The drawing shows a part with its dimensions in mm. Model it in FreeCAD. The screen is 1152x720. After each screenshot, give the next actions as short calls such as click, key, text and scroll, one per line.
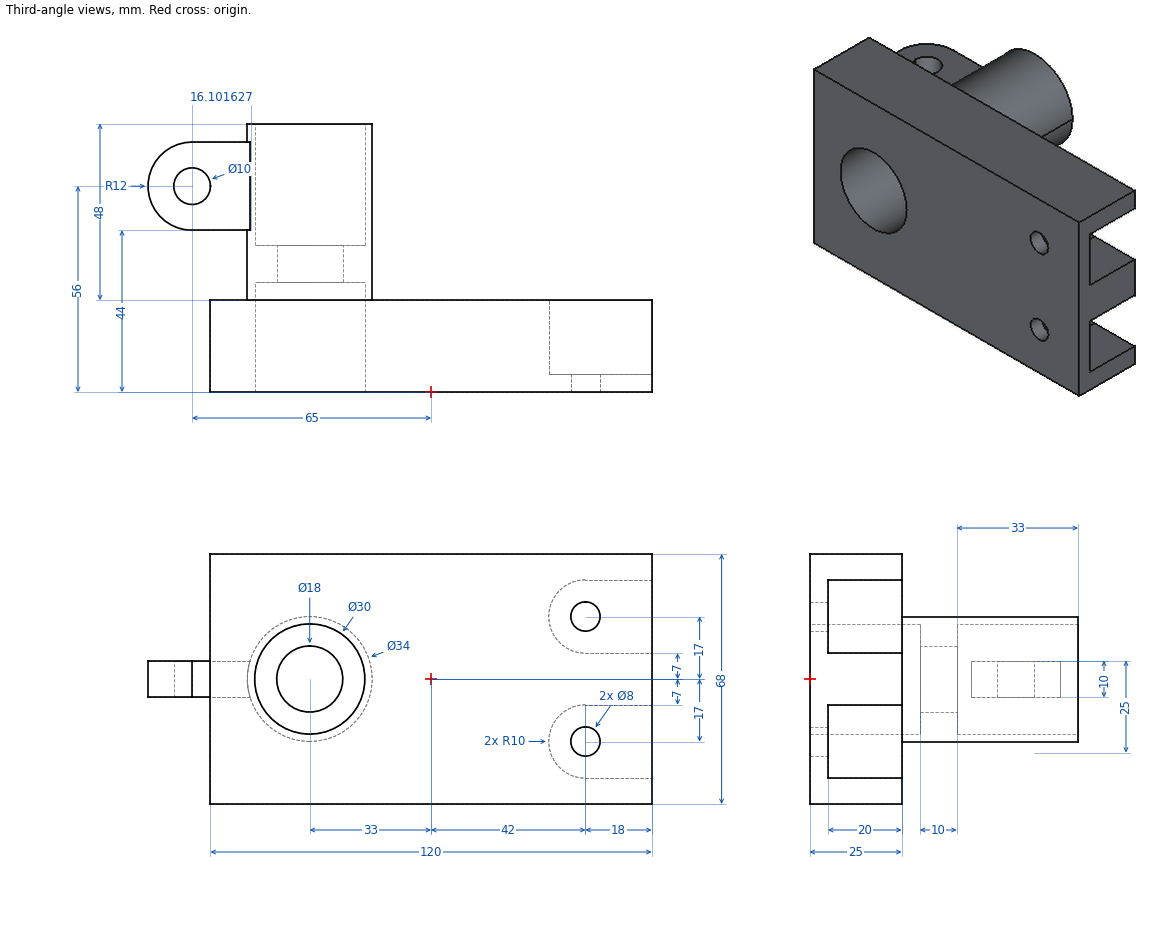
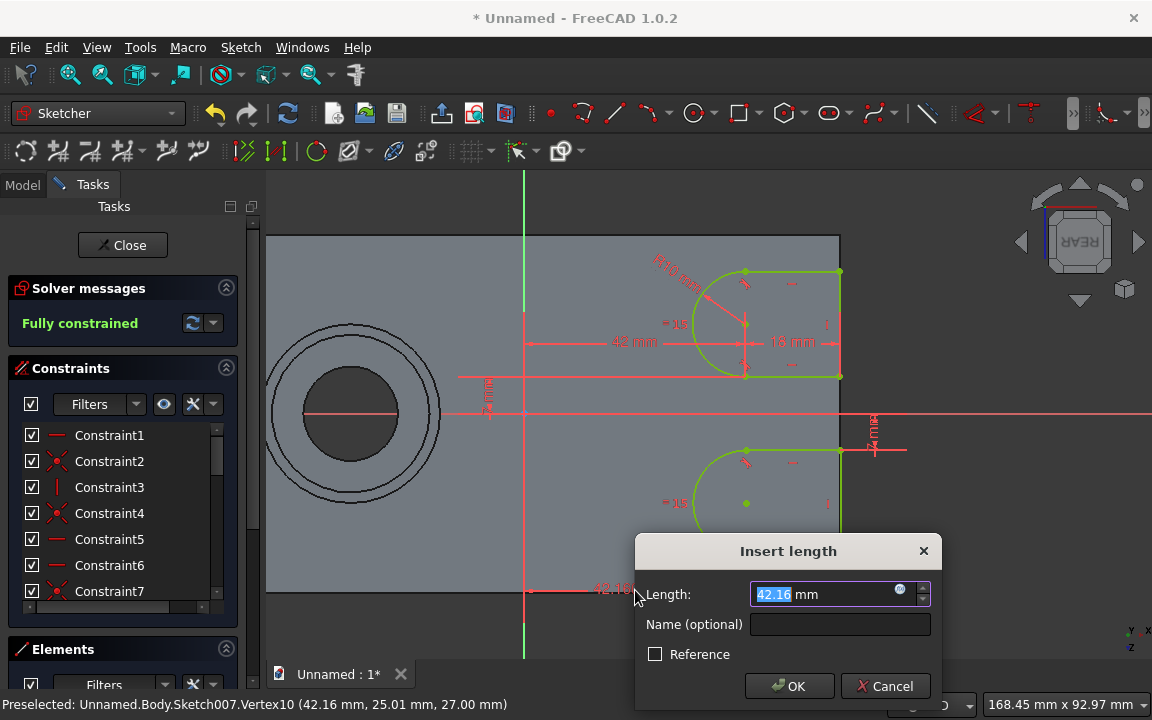
text(42)
key(Return)
key(Escape)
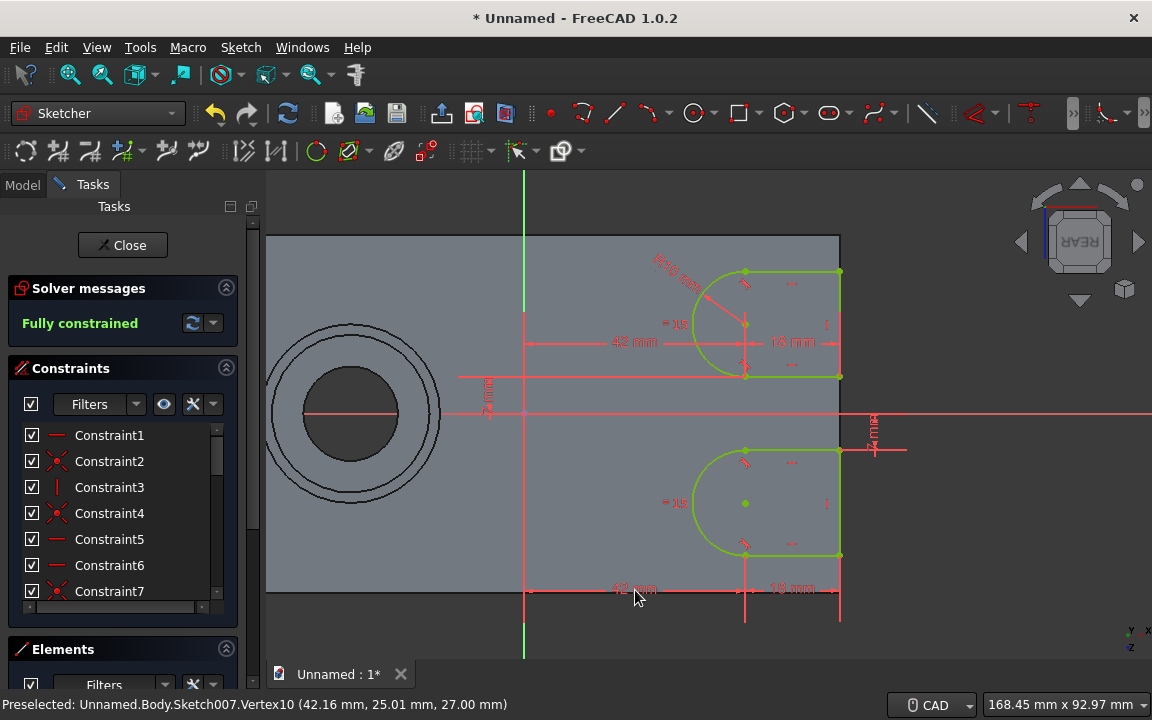
click(123, 245)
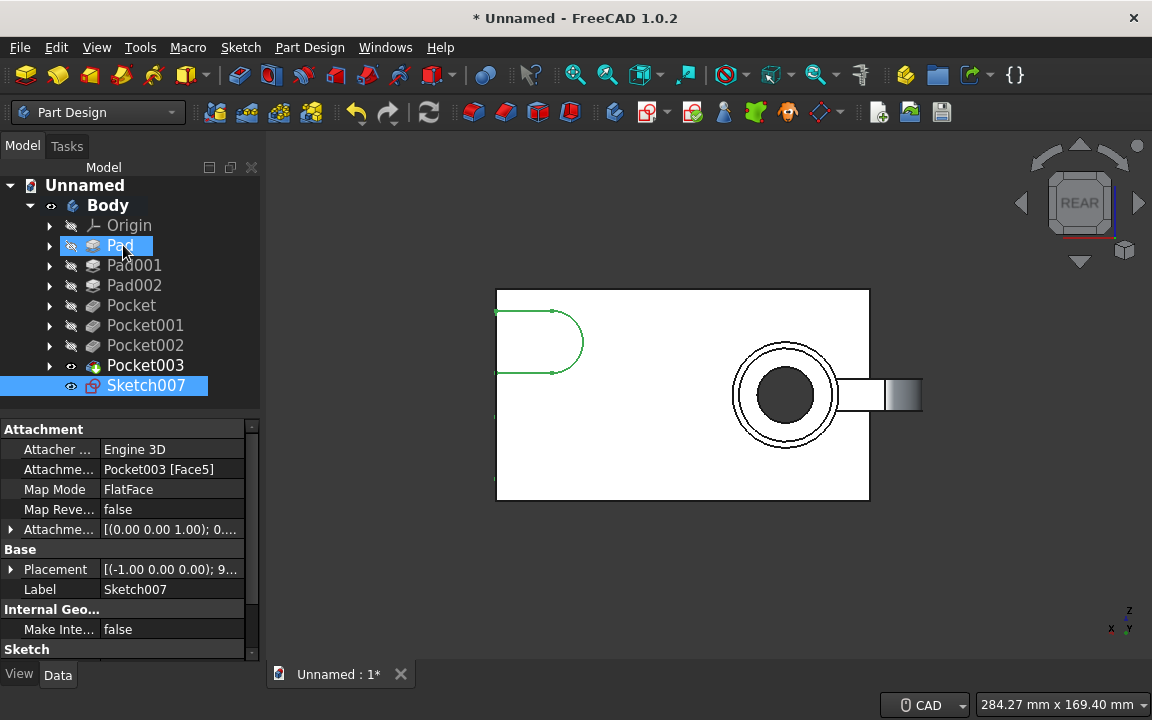
click(240, 76)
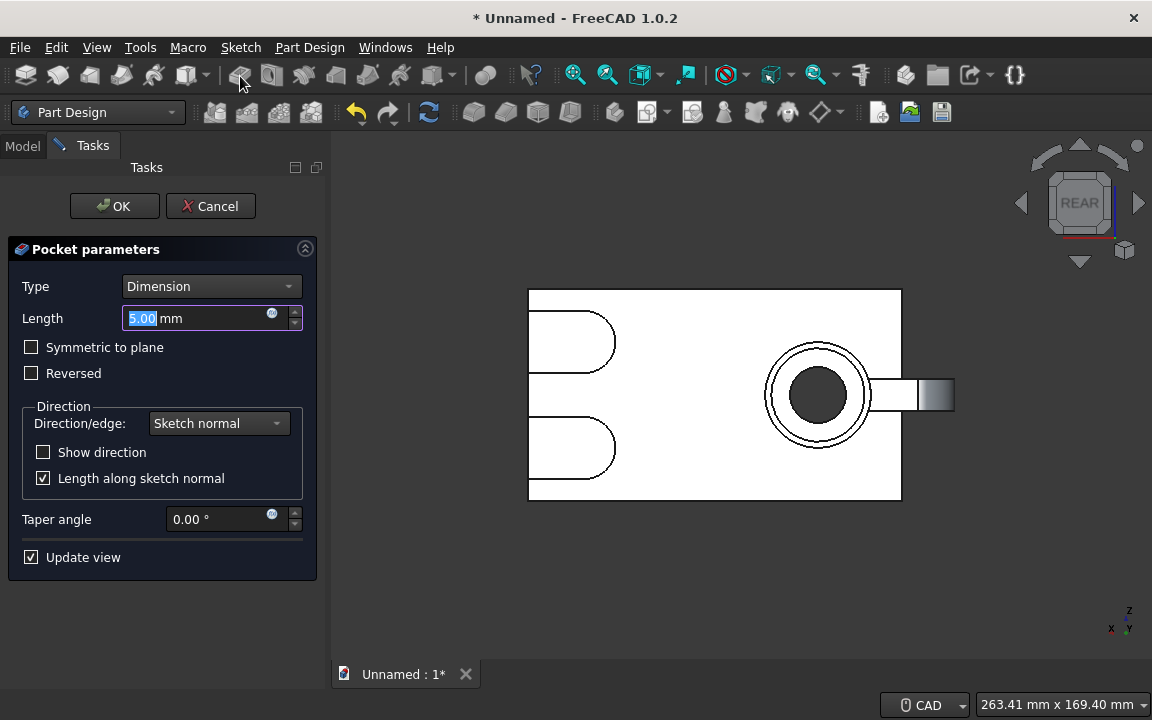
text(20)
key(Tab)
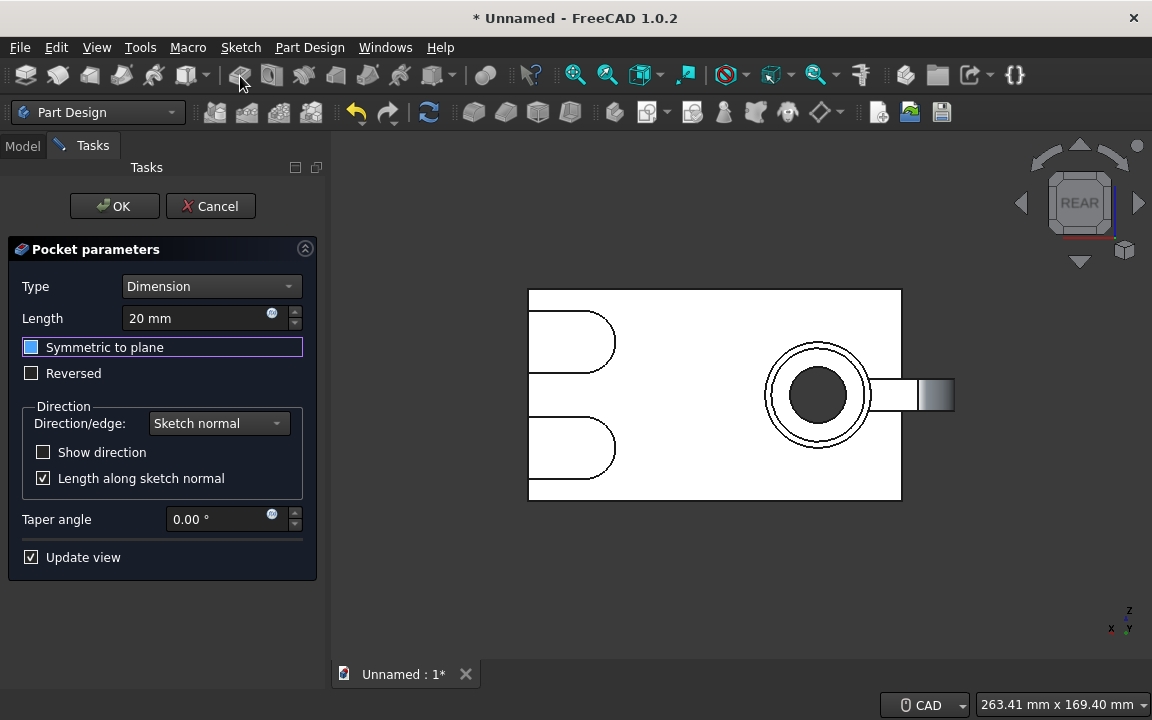
click(115, 206)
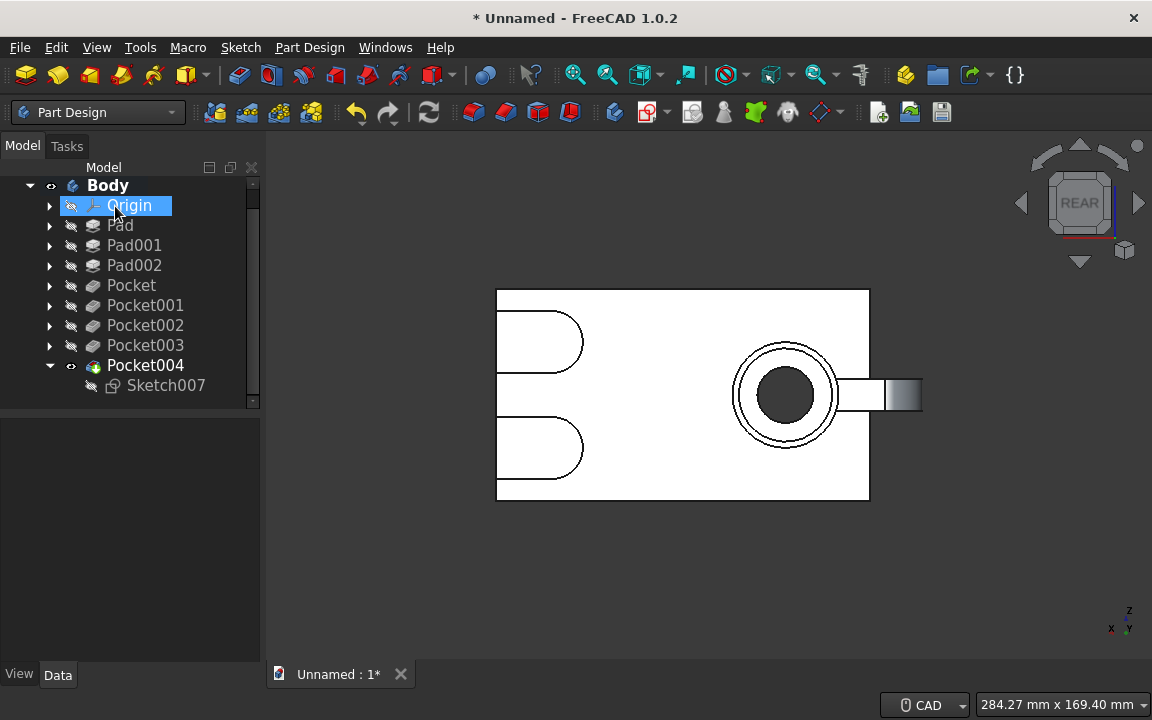
click(539, 341)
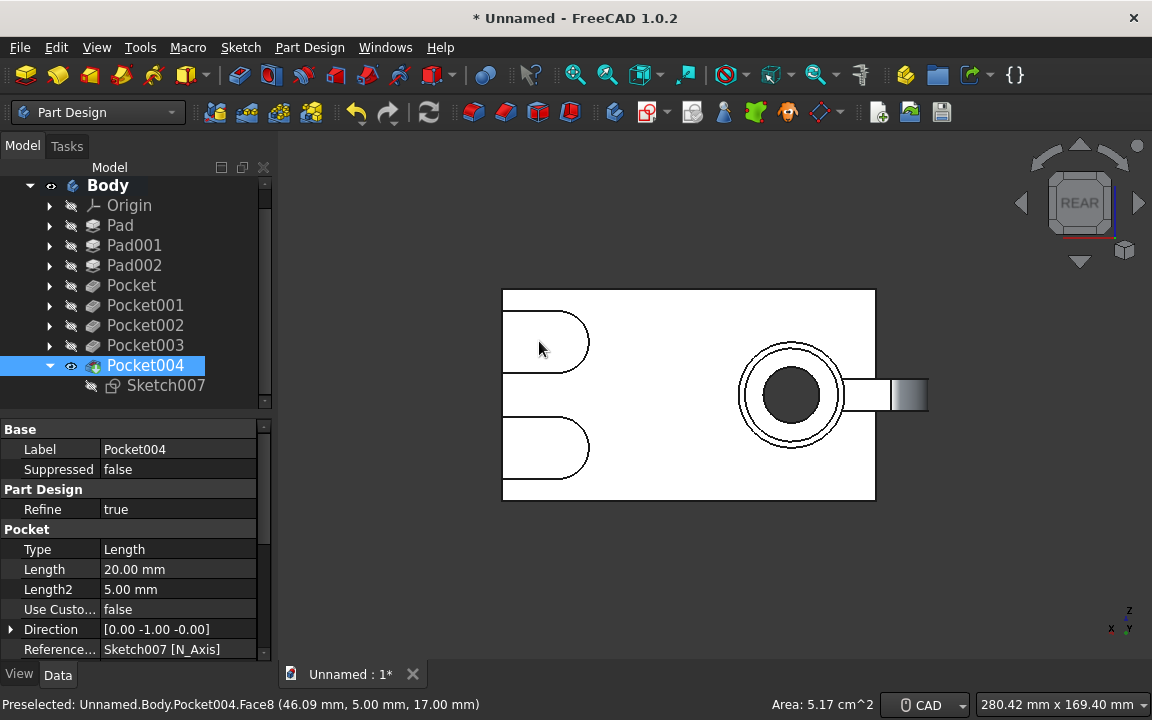
click(648, 112)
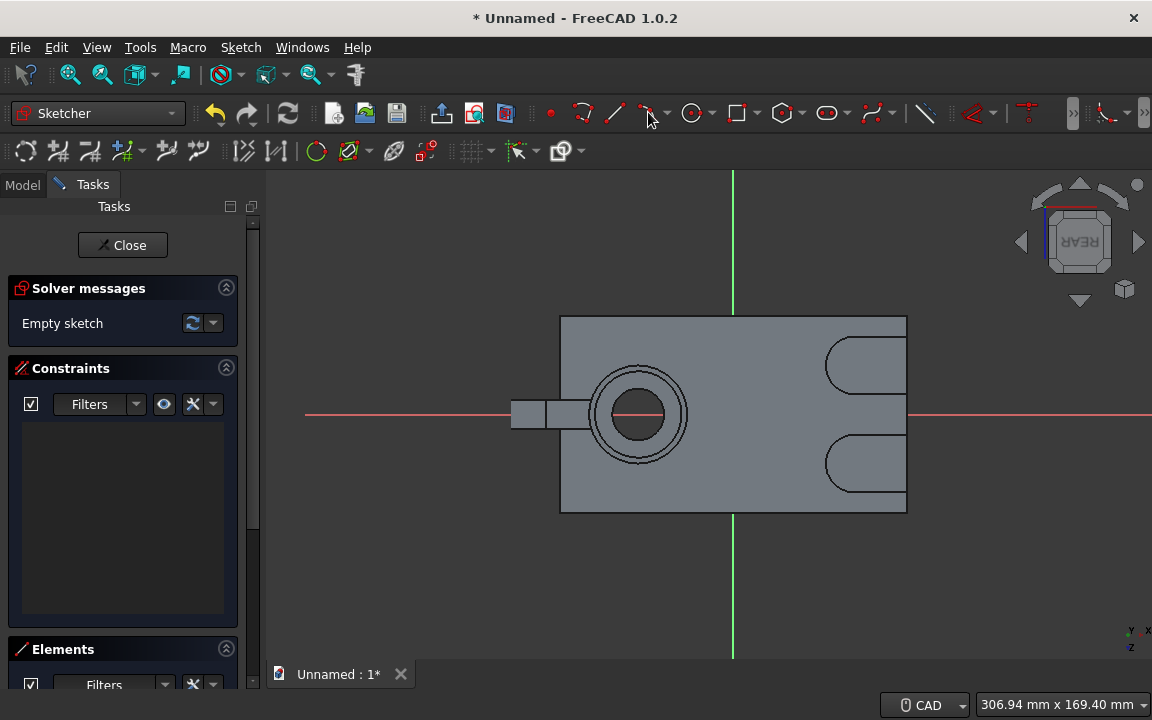
scroll(893, 414, up, 5)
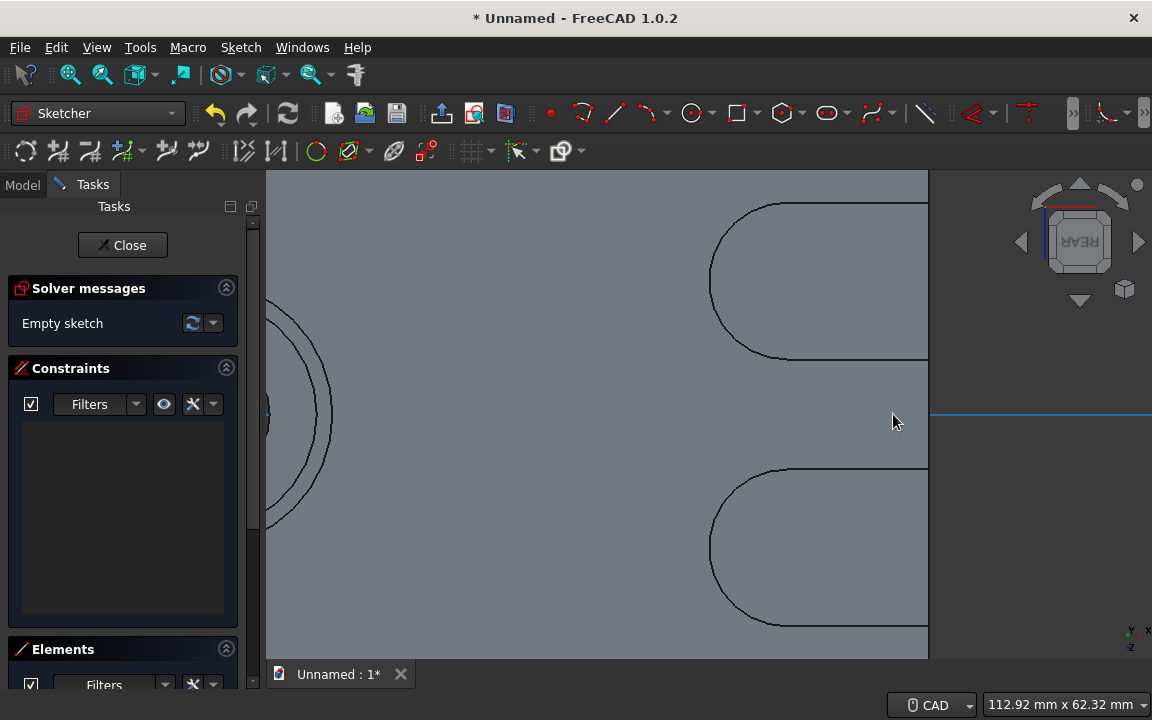
click(692, 114)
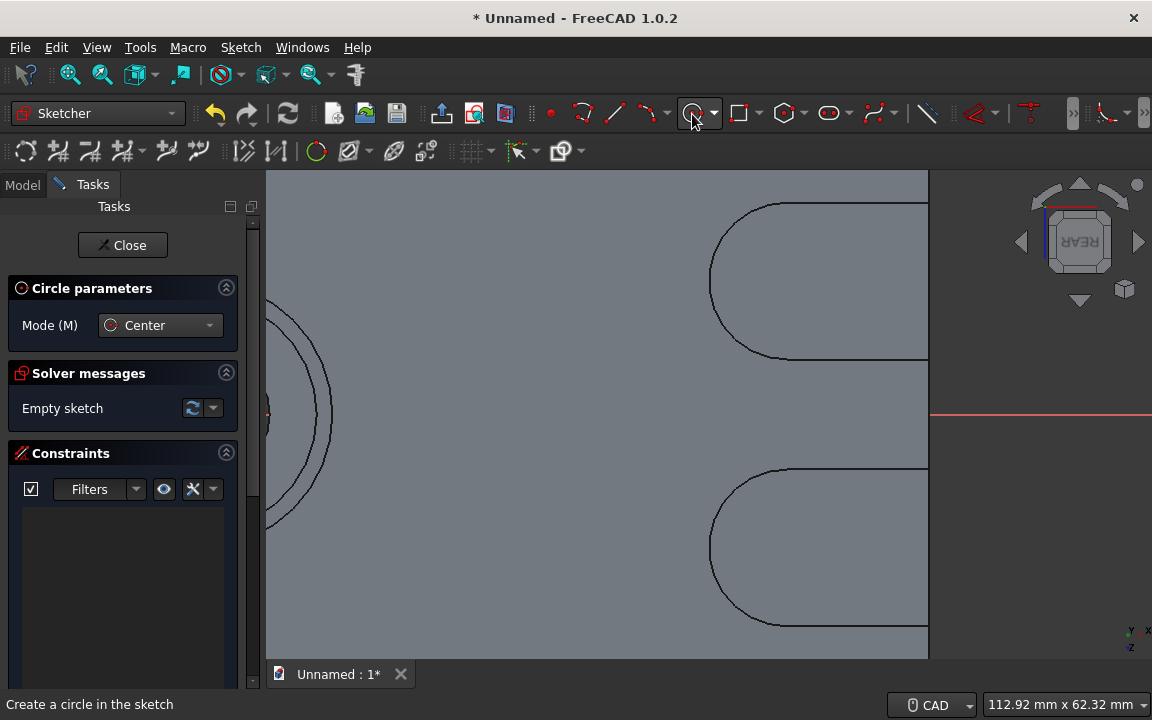
click(788, 281)
move(810, 259)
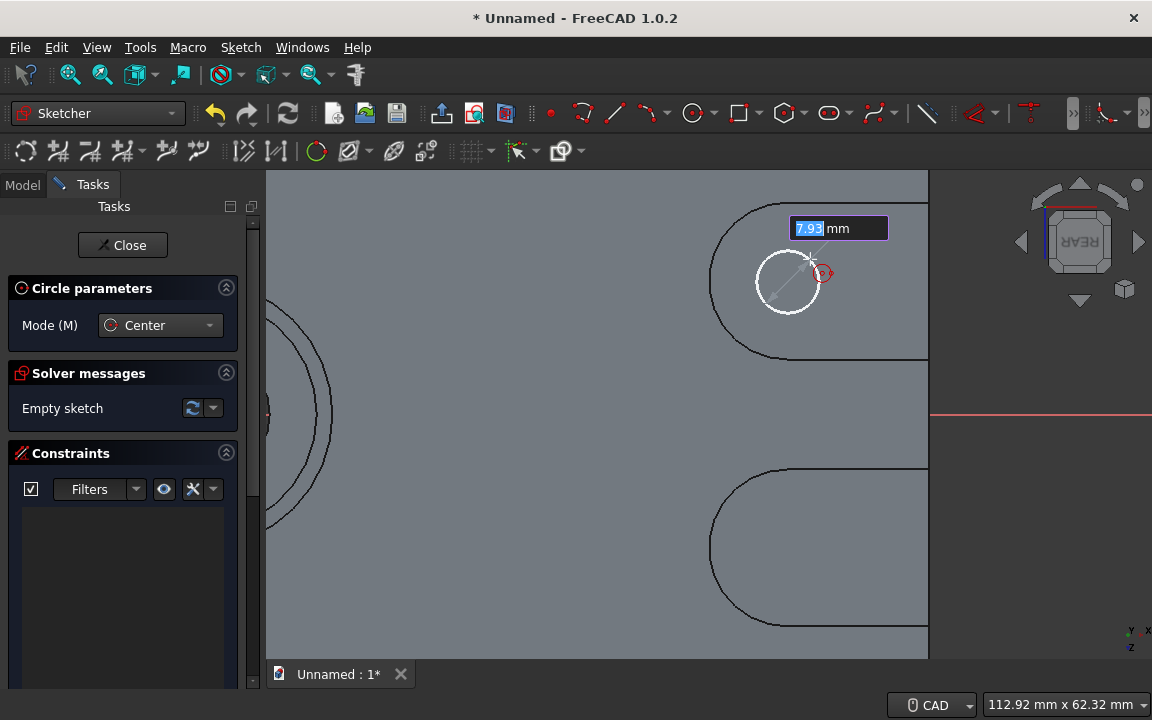
text(8)
key(Return)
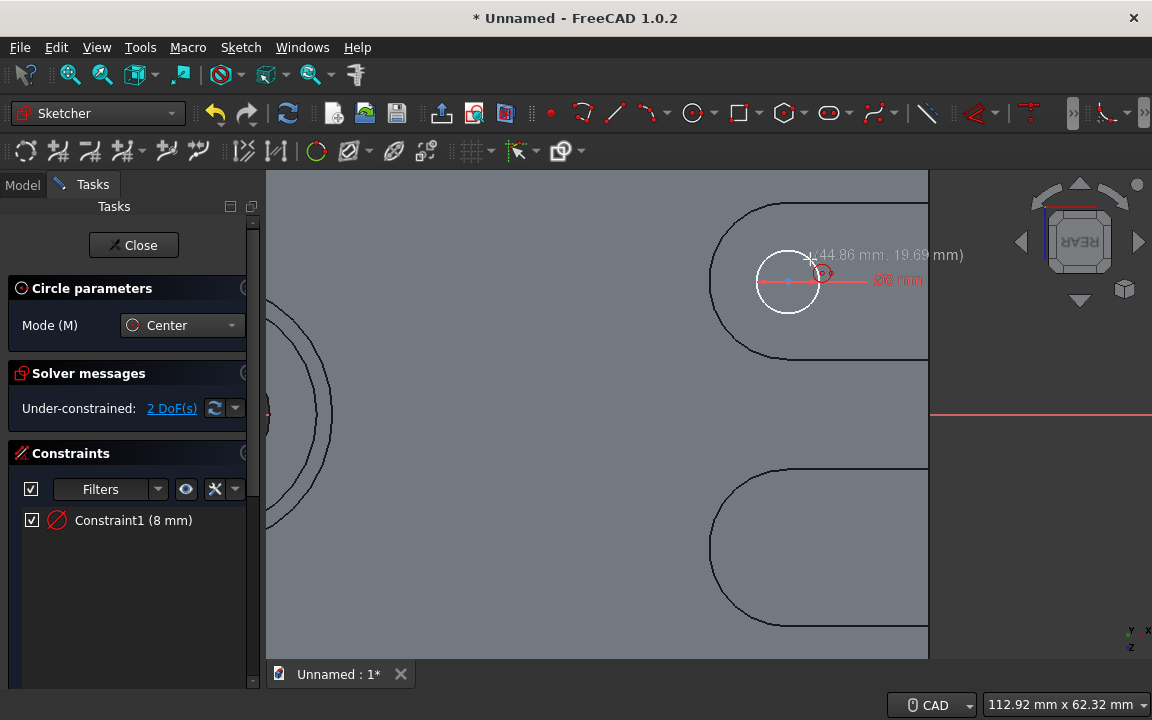
click(788, 548)
move(810, 526)